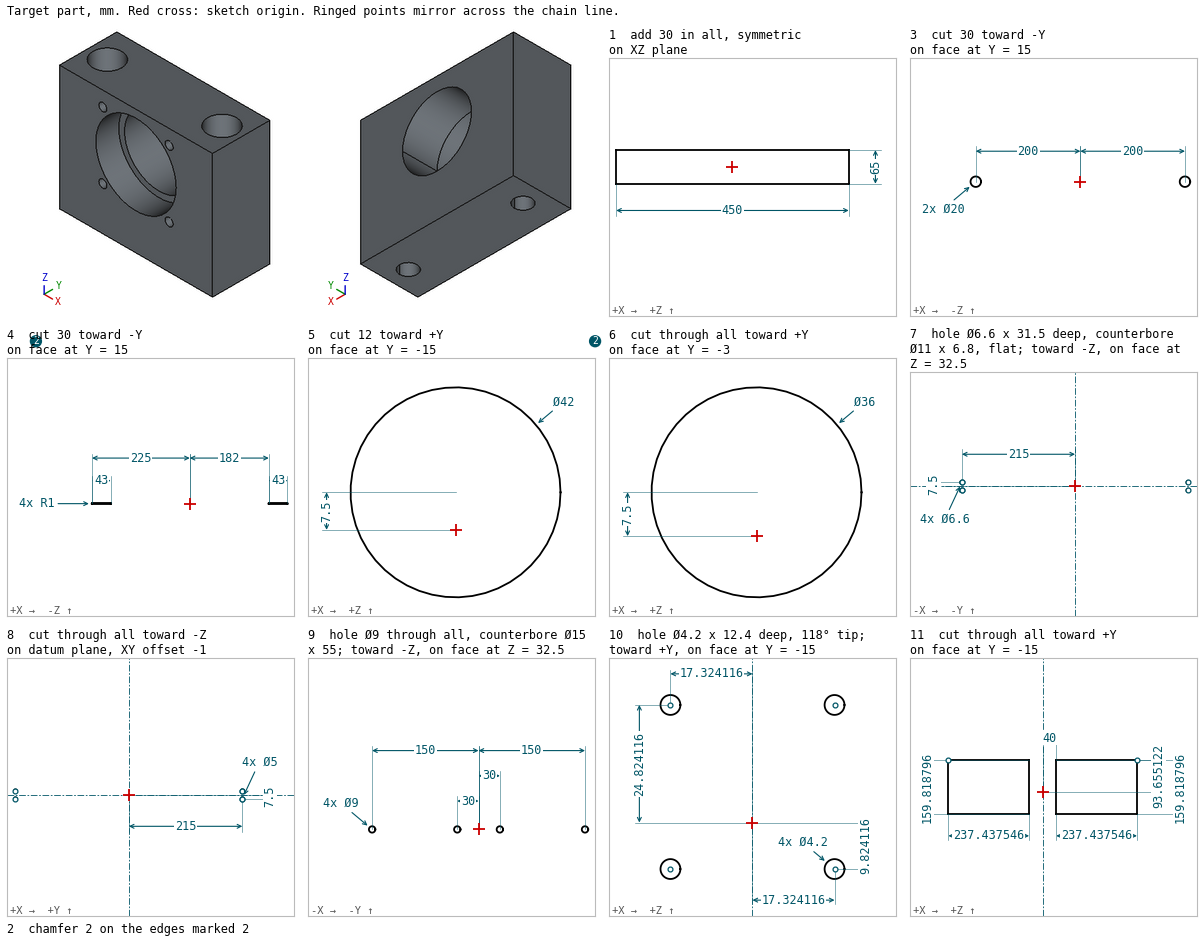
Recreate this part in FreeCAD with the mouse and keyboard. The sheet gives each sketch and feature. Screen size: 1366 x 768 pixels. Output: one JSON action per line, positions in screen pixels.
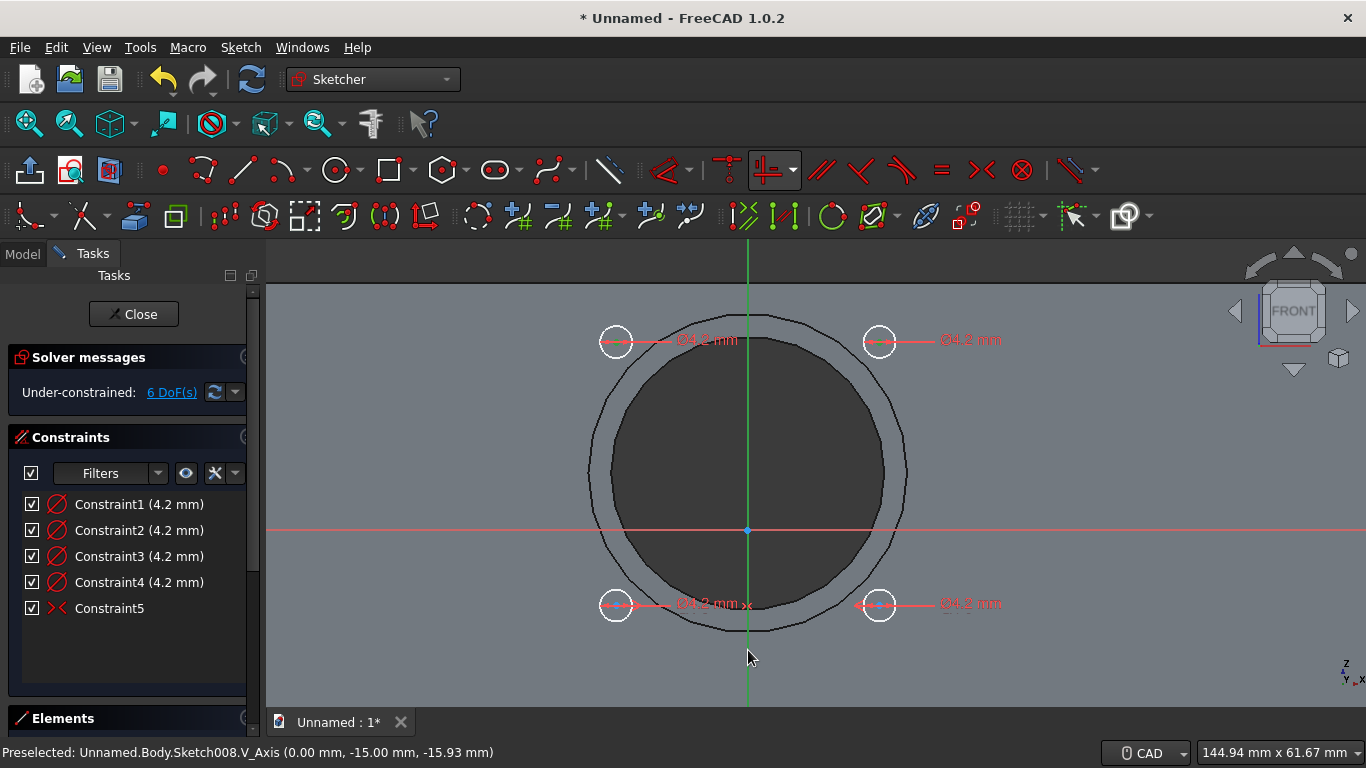
{"action": "left_click", "coordinate": [982, 170]}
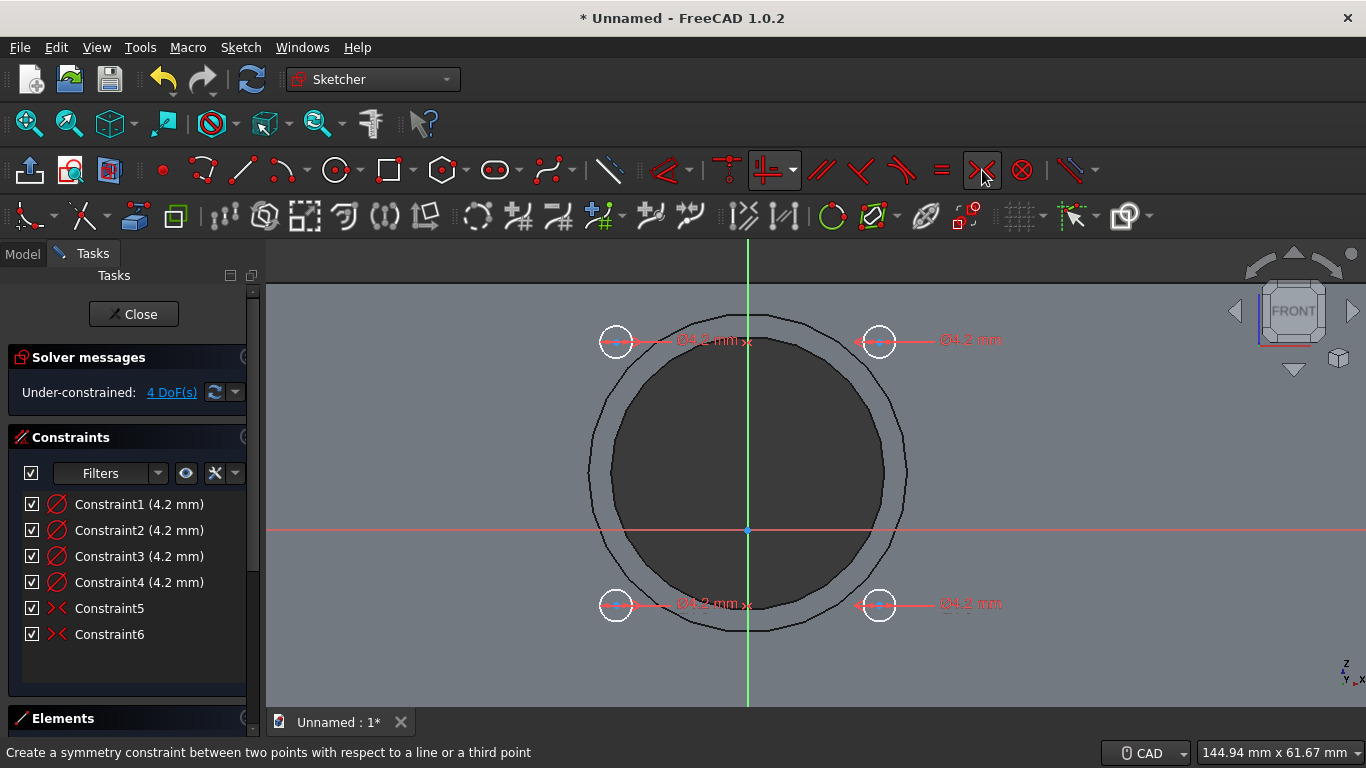
{"action": "key", "text": "d"}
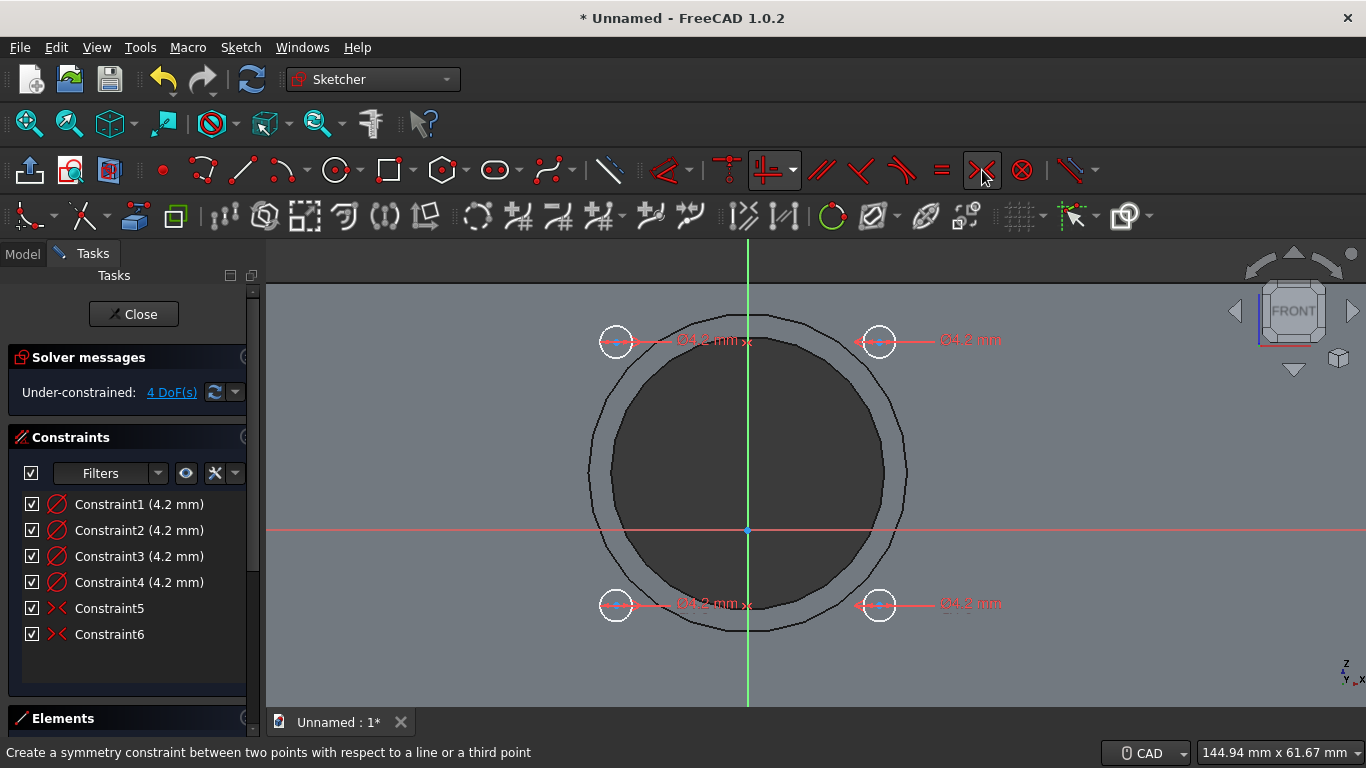
{"action": "left_click", "coordinate": [879, 606]}
{"action": "left_click", "coordinate": [913, 568]}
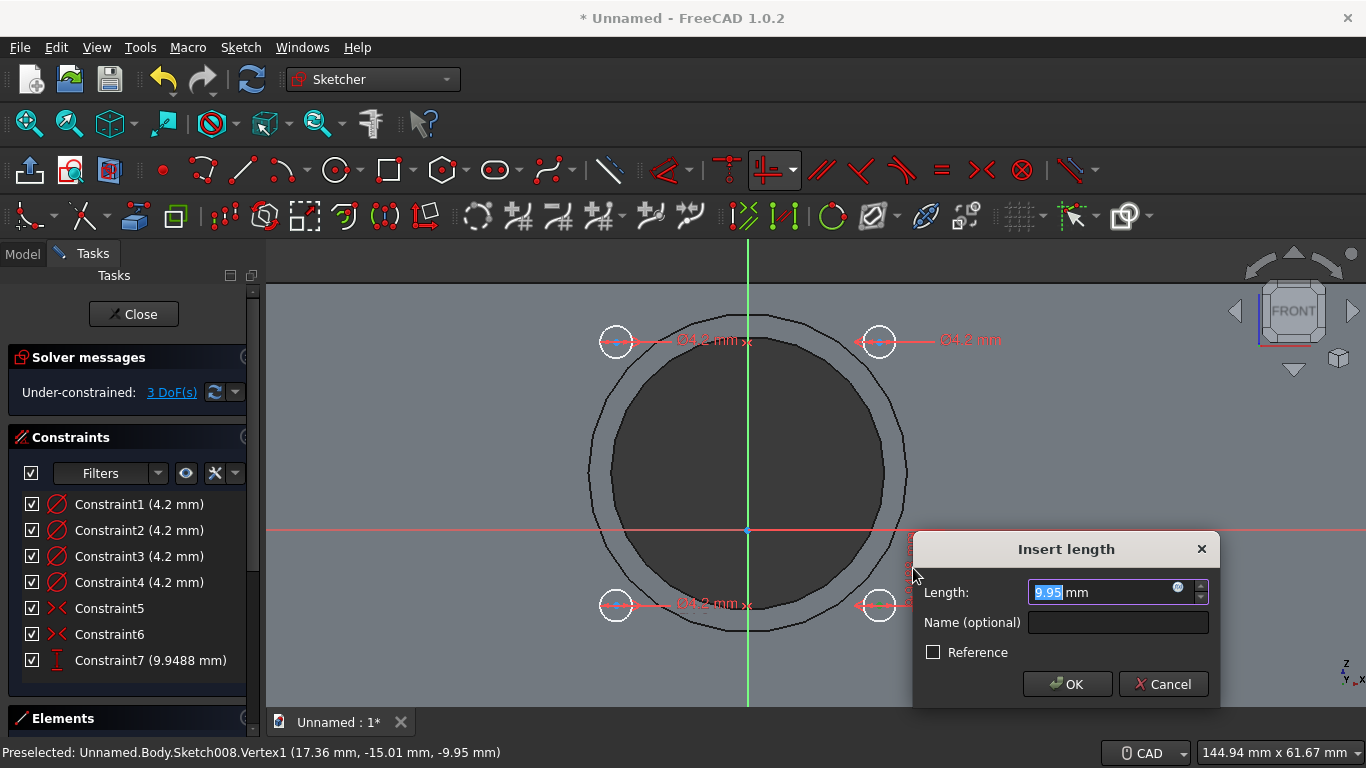
{"action": "type", "text": "9.824116"}
{"action": "key", "text": "Return"}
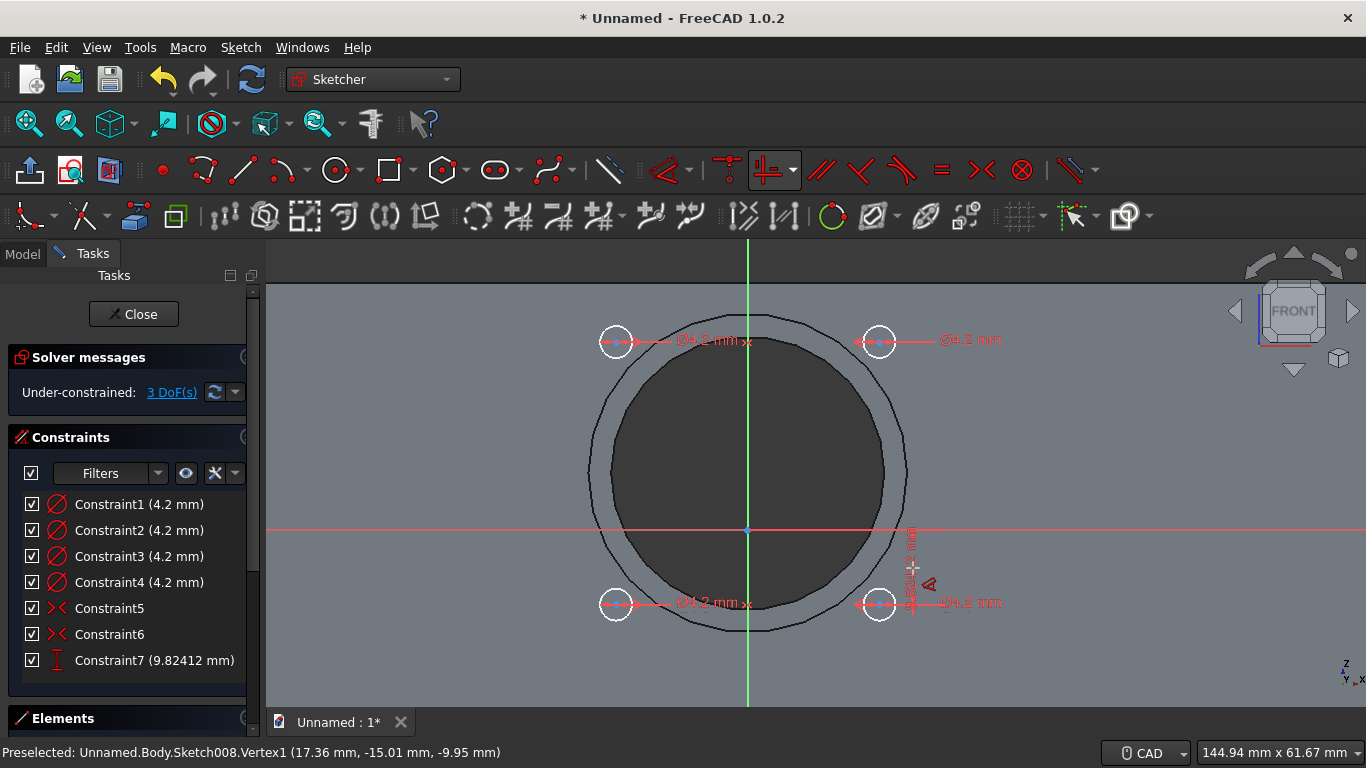
{"action": "left_click", "coordinate": [879, 605]}
{"action": "left_click", "coordinate": [814, 639]}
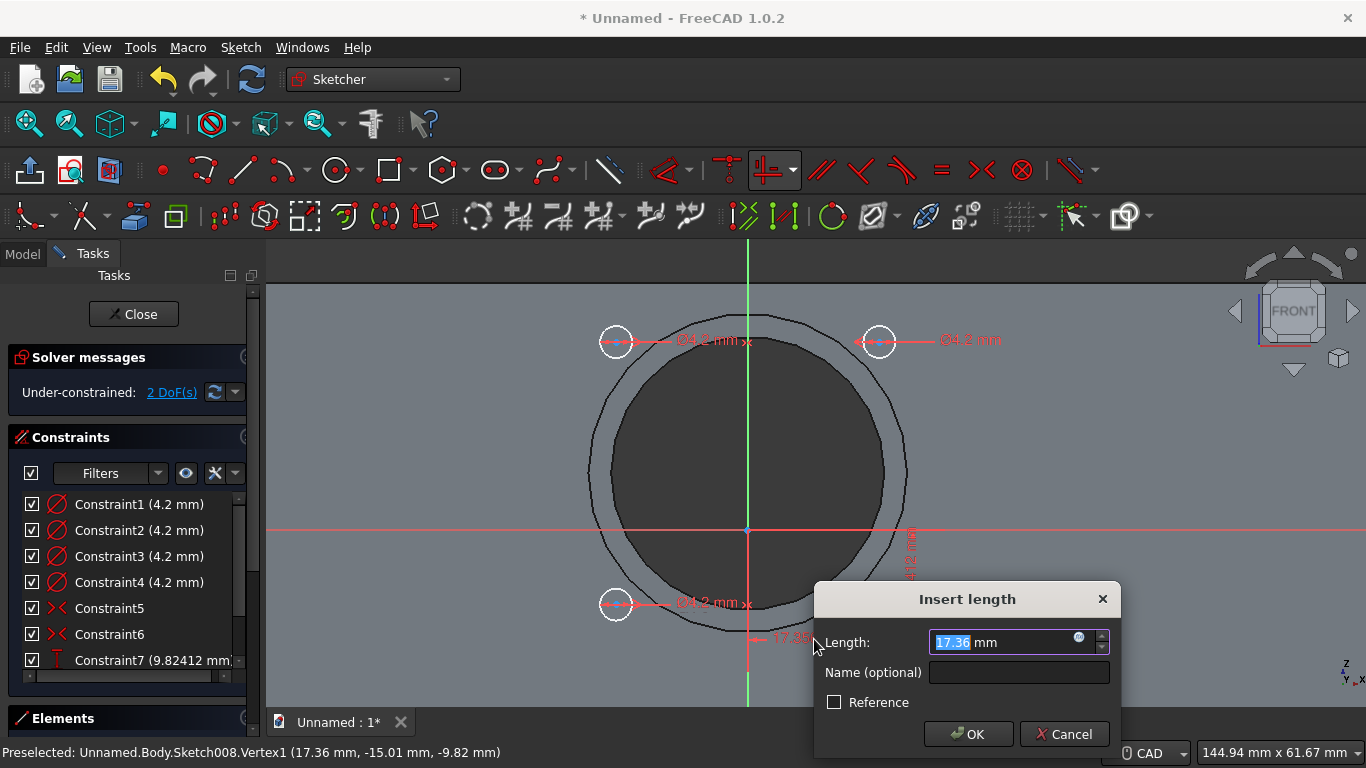
{"action": "type", "text": "17.324116"}
{"action": "key", "text": "Return"}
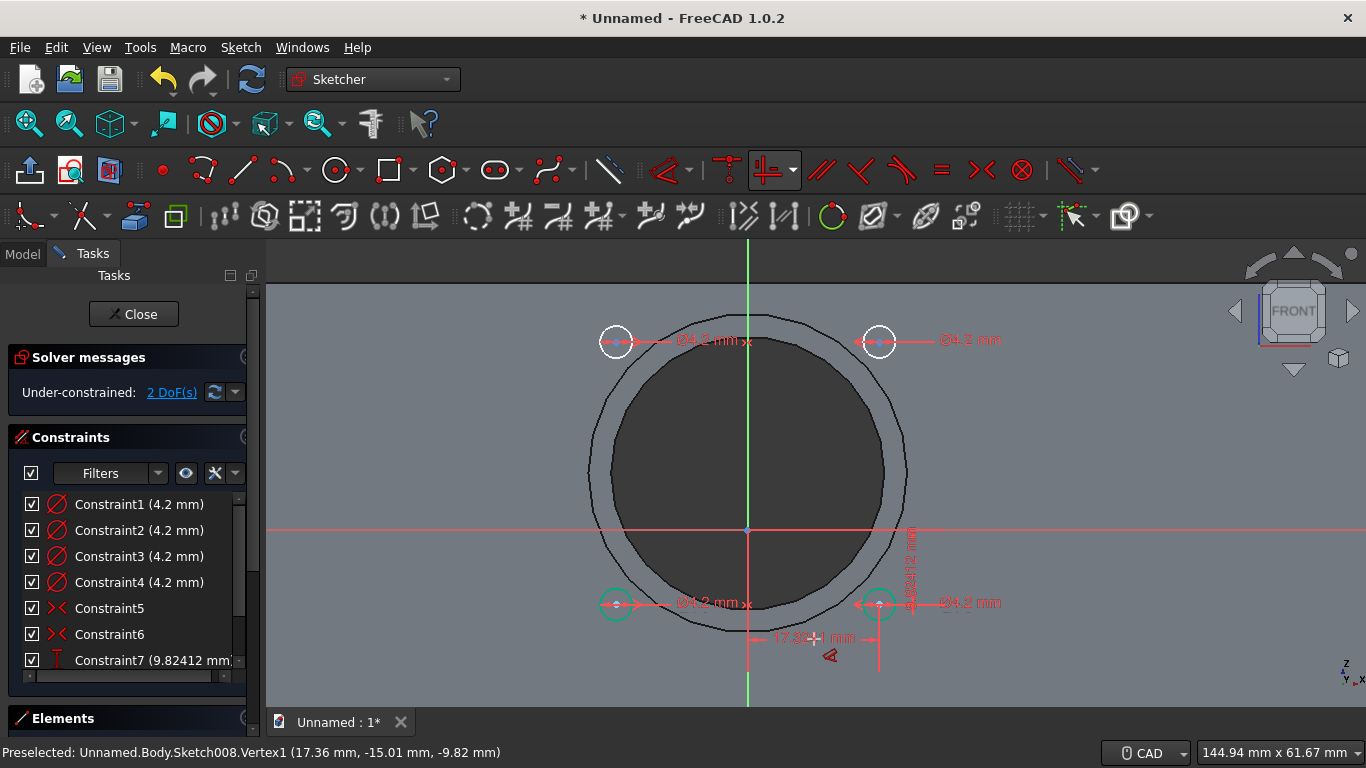
{"action": "left_click", "coordinate": [616, 342]}
{"action": "left_click", "coordinate": [682, 308]}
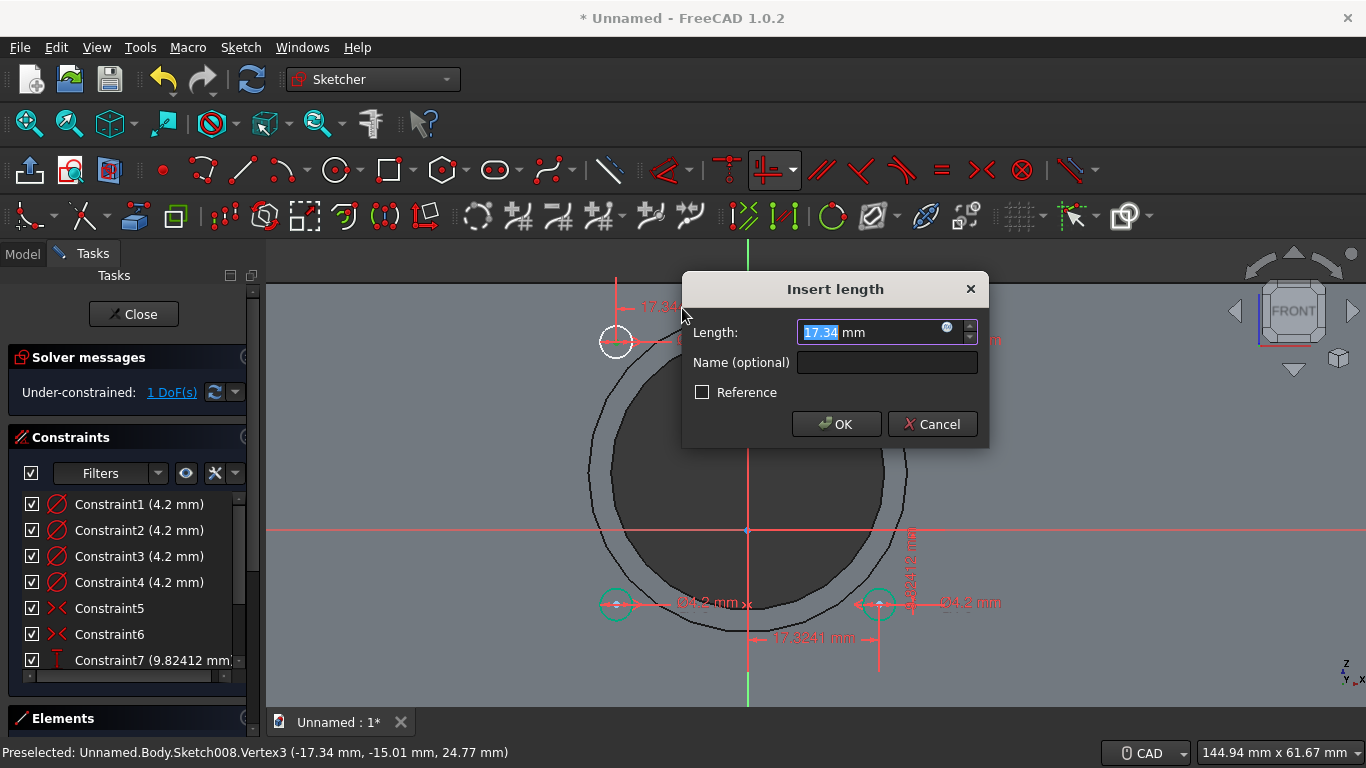
{"action": "type", "text": "17.324116"}
{"action": "key", "text": "Return"}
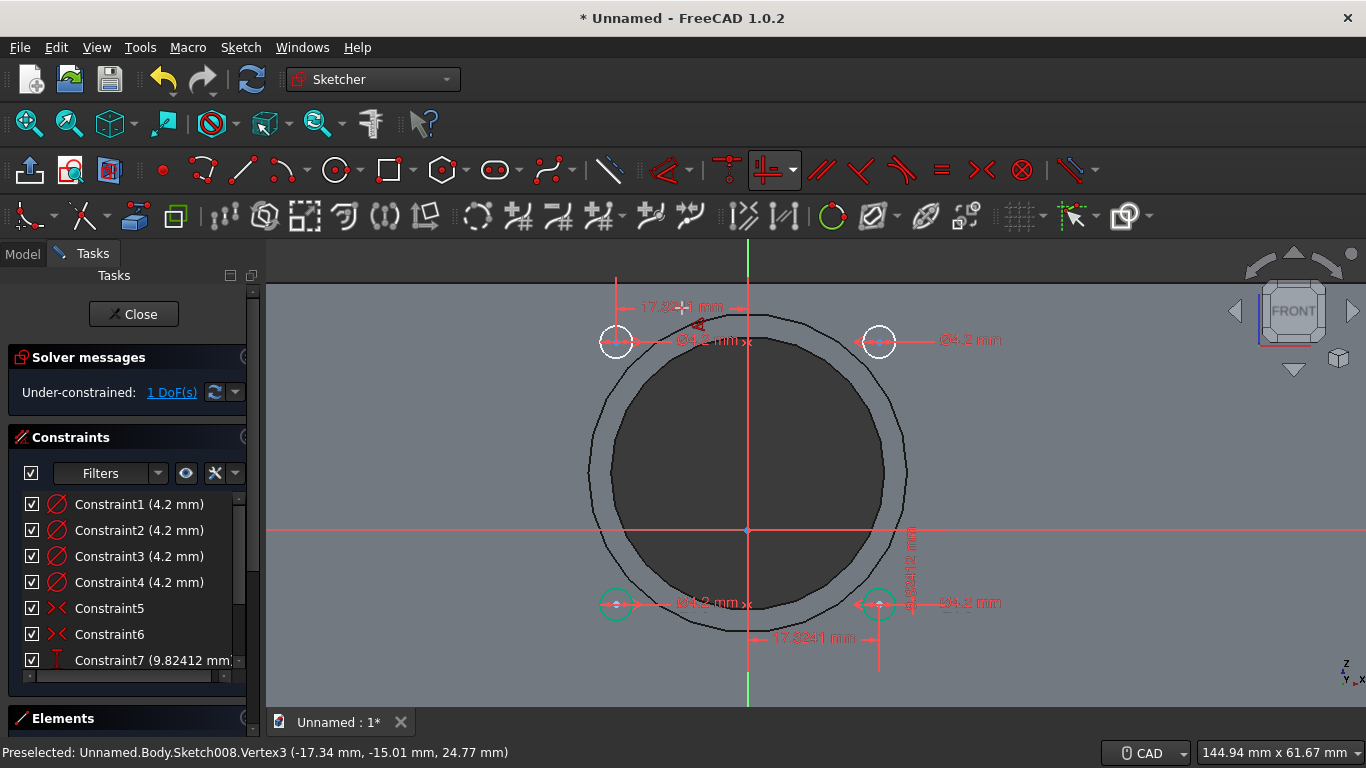
{"action": "left_click", "coordinate": [616, 342]}
{"action": "left_click", "coordinate": [582, 436]}